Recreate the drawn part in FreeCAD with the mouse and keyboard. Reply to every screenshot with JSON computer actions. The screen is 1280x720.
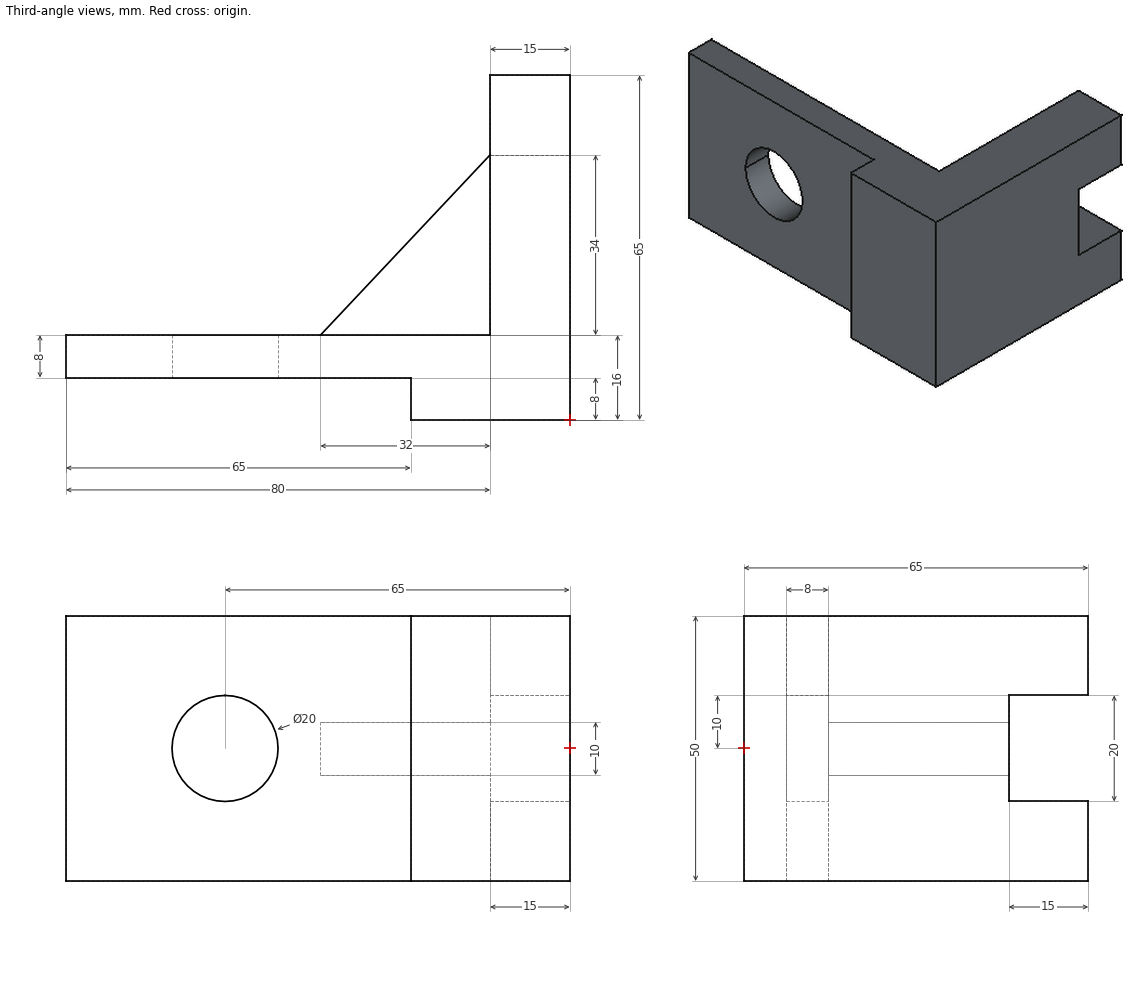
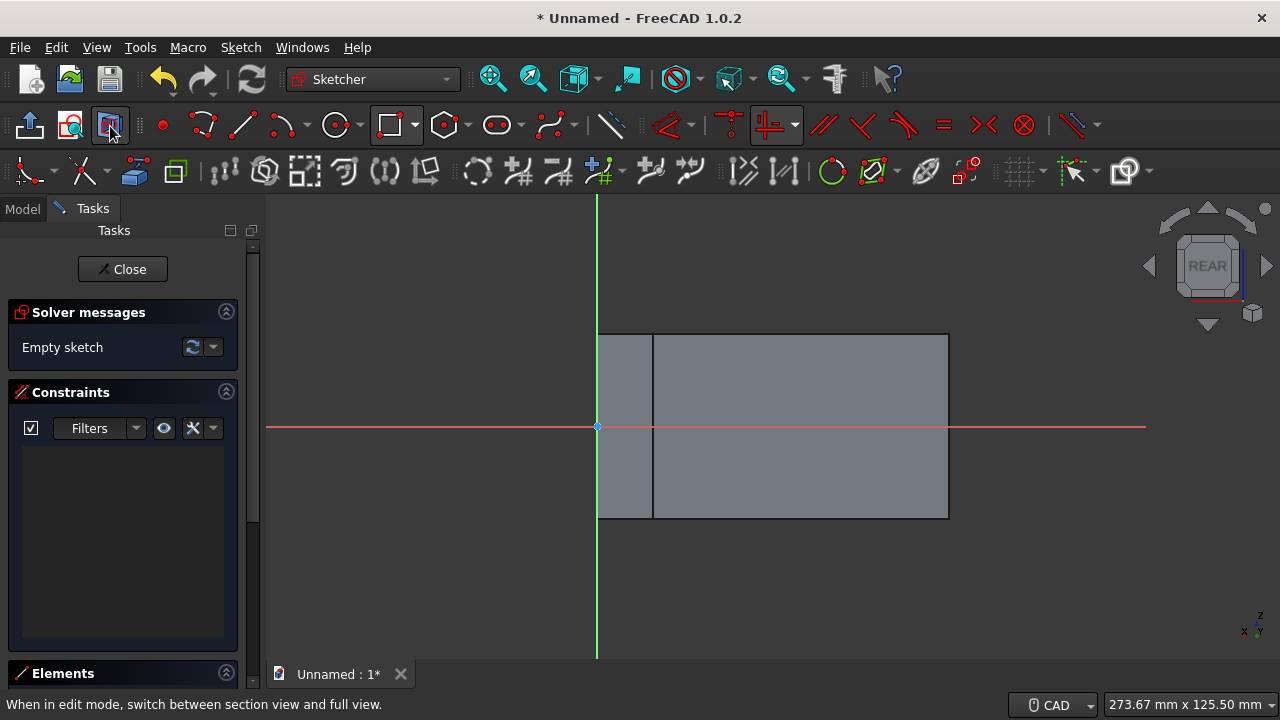
{"action": "scroll", "coordinate": [881, 426], "scroll_direction": "up", "scroll_amount": 7}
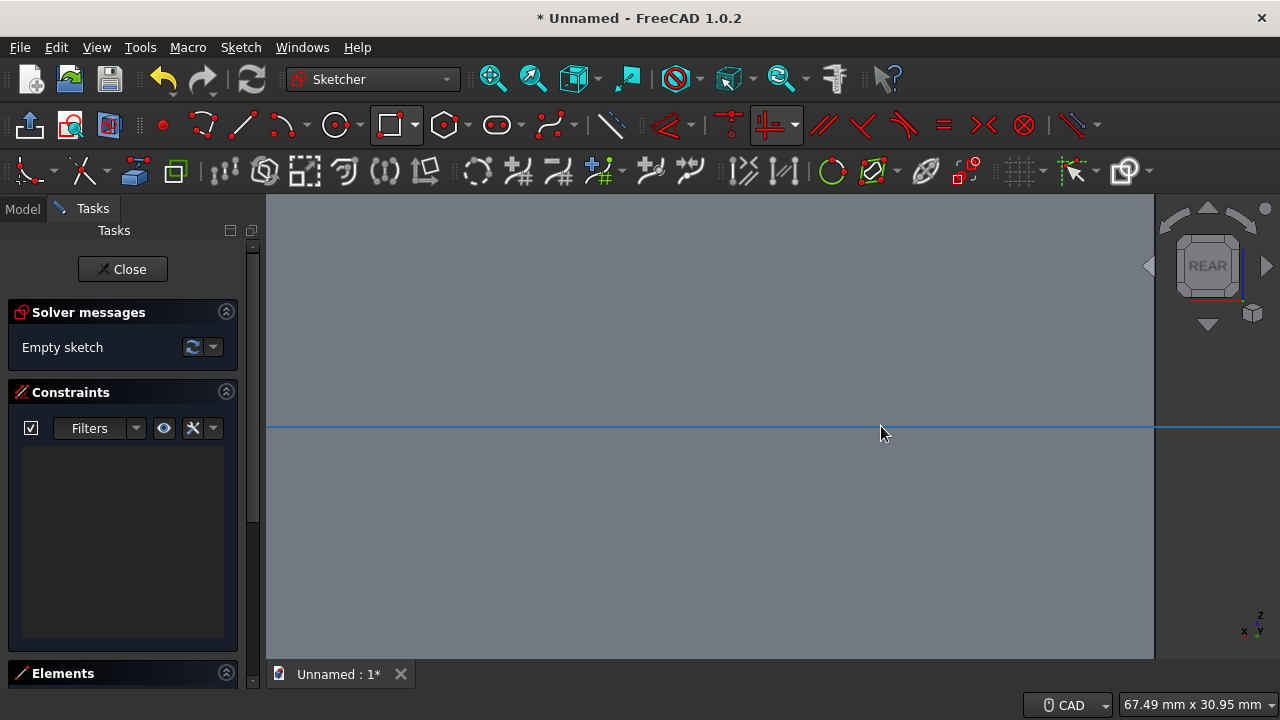
{"action": "key", "text": "g c"}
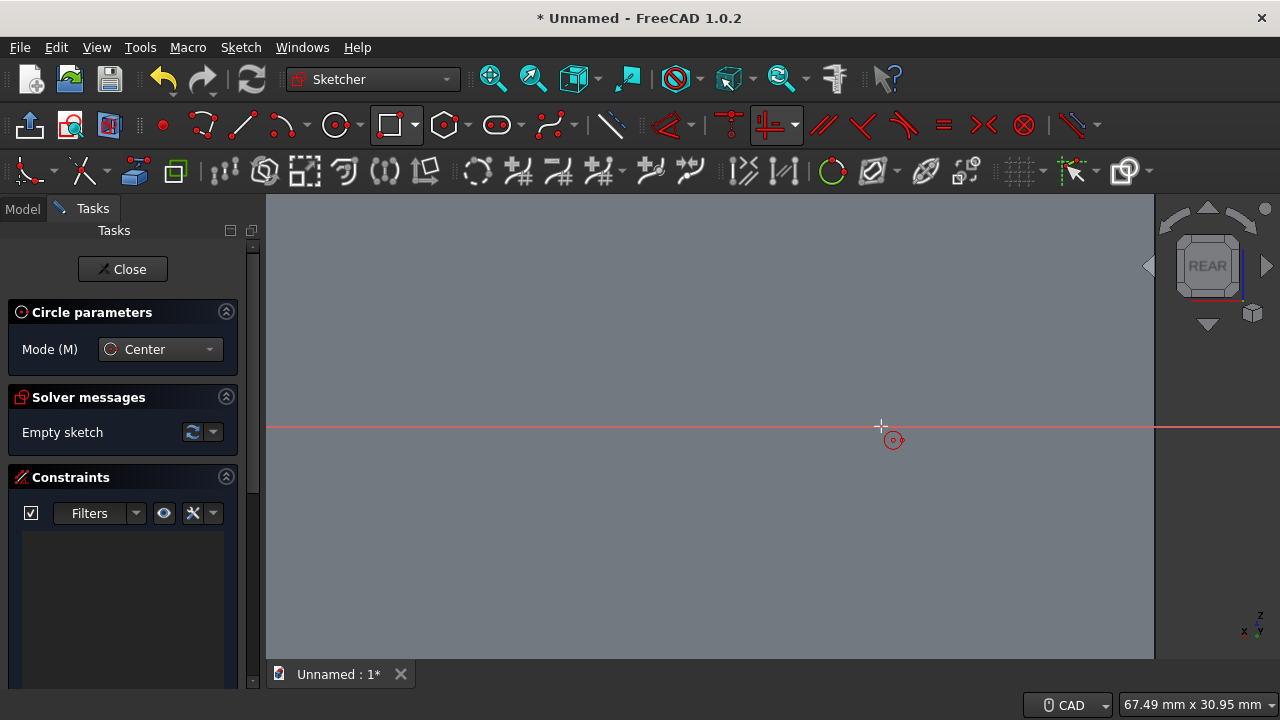
{"action": "left_click", "coordinate": [704, 426]}
{"action": "mouse_move", "coordinate": [810, 320]}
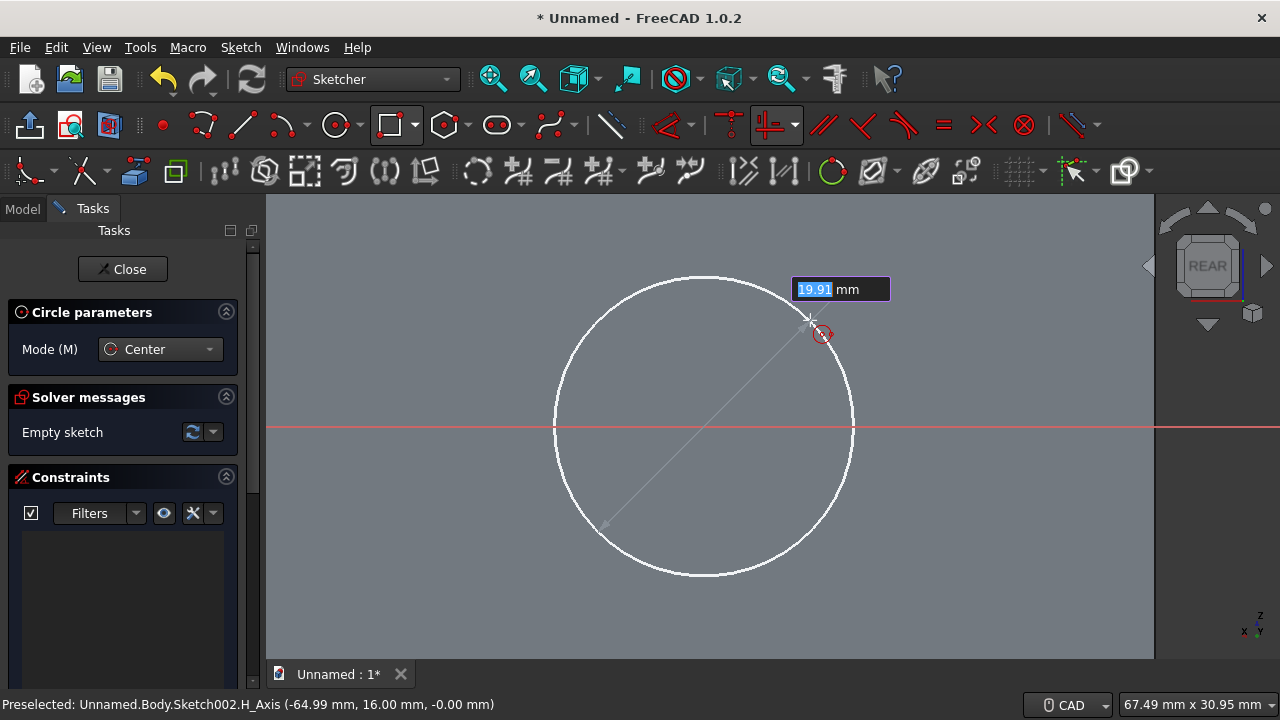
{"action": "type", "text": "20"}
{"action": "key", "text": "Return"}
{"action": "key", "text": "Escape"}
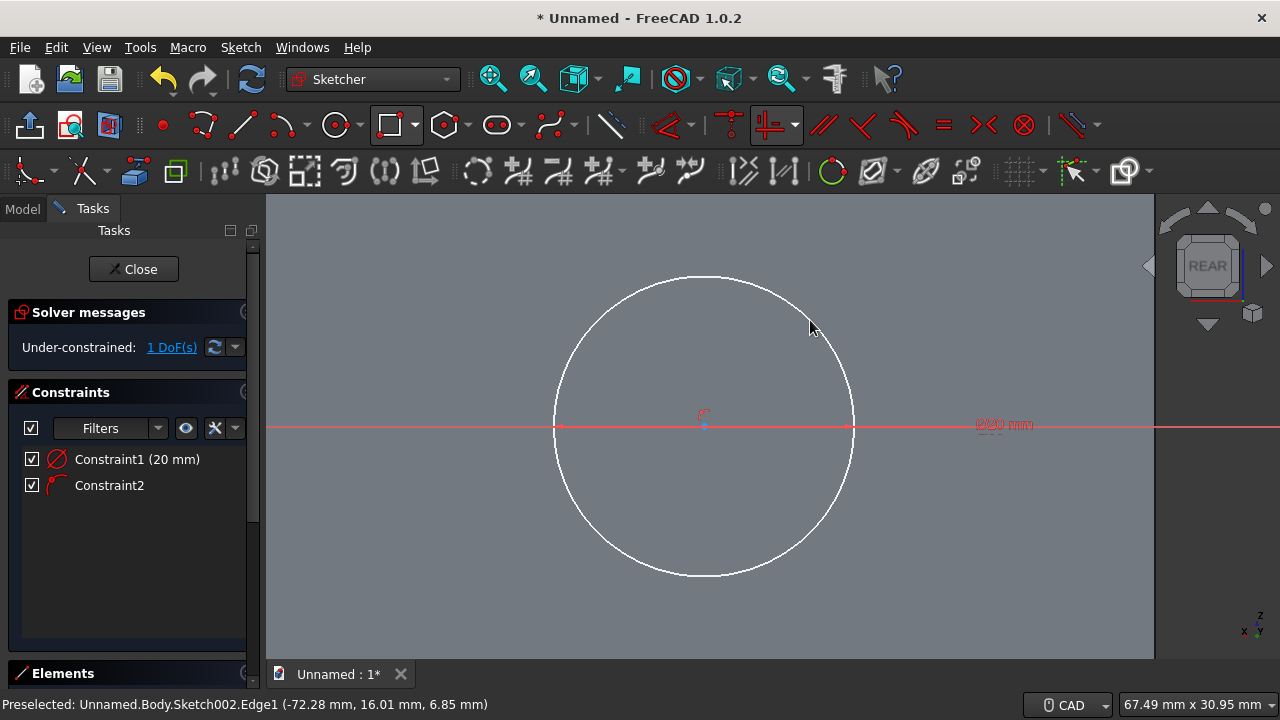
{"action": "key", "text": "d"}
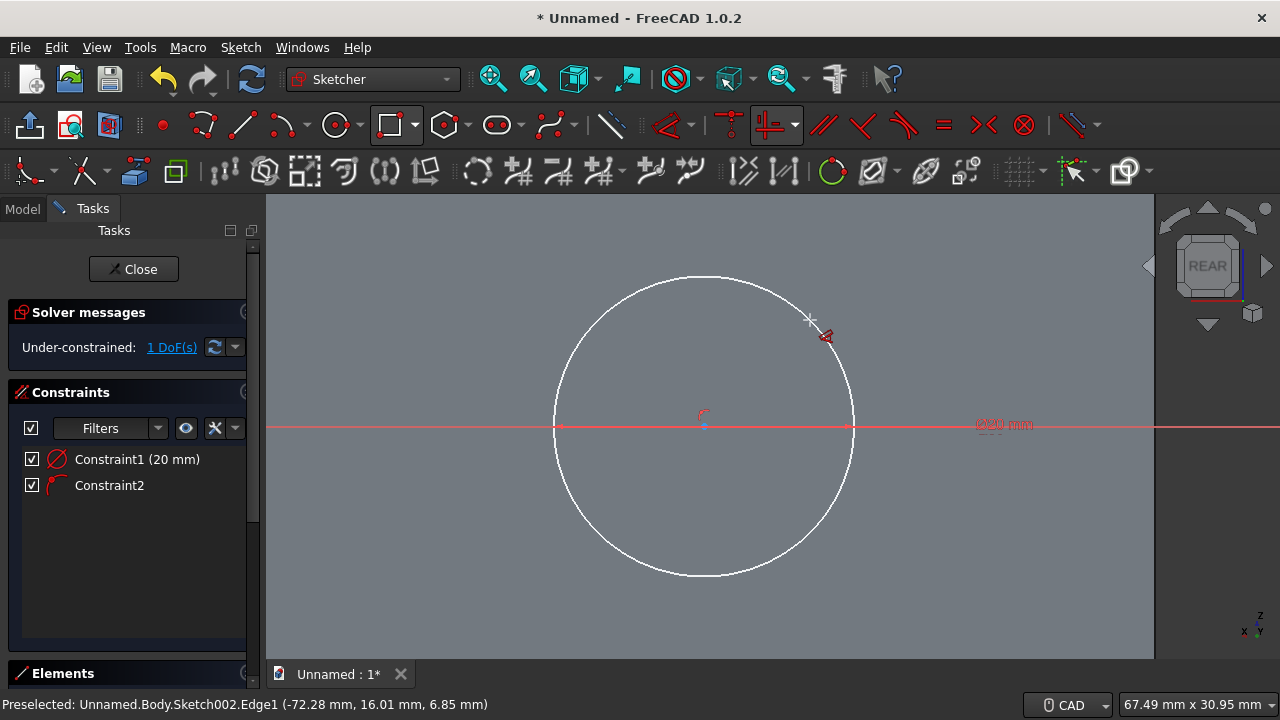
{"action": "left_click", "coordinate": [704, 426]}
{"action": "left_click", "coordinate": [499, 460]}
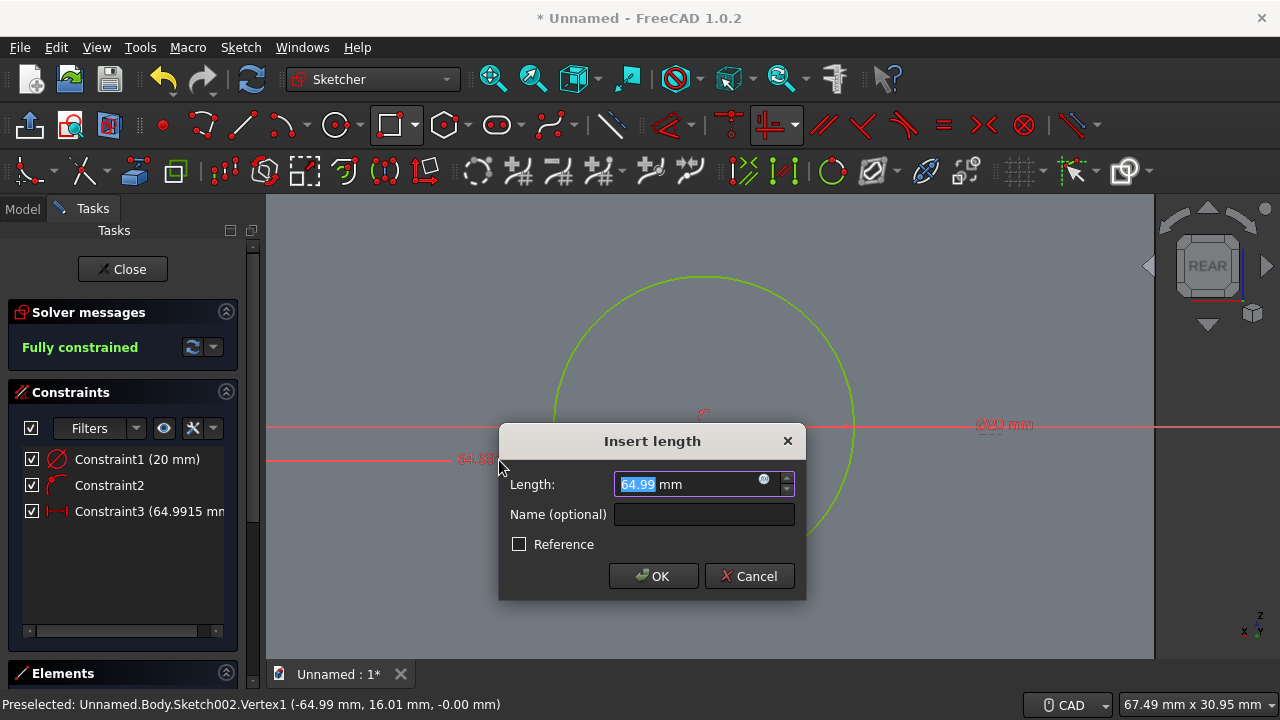
{"action": "type", "text": "65"}
{"action": "key", "text": "Return"}
{"action": "key", "text": "Escape"}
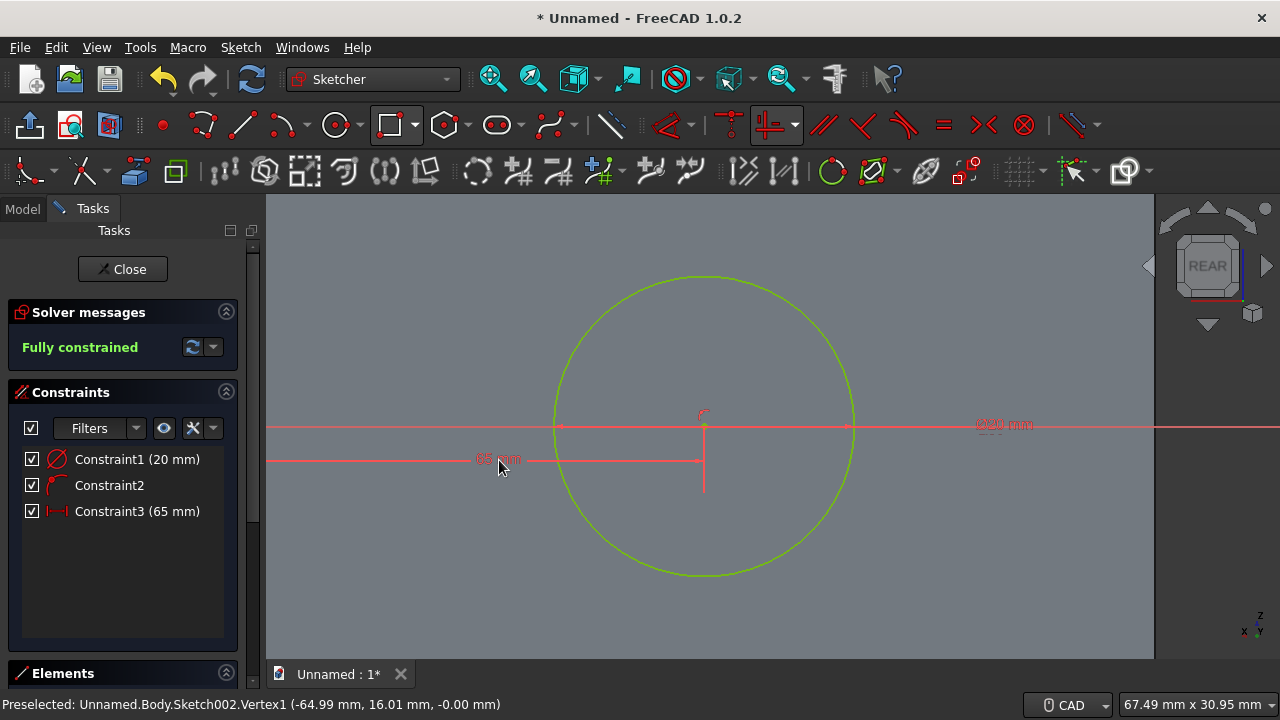
{"action": "left_click", "coordinate": [123, 269]}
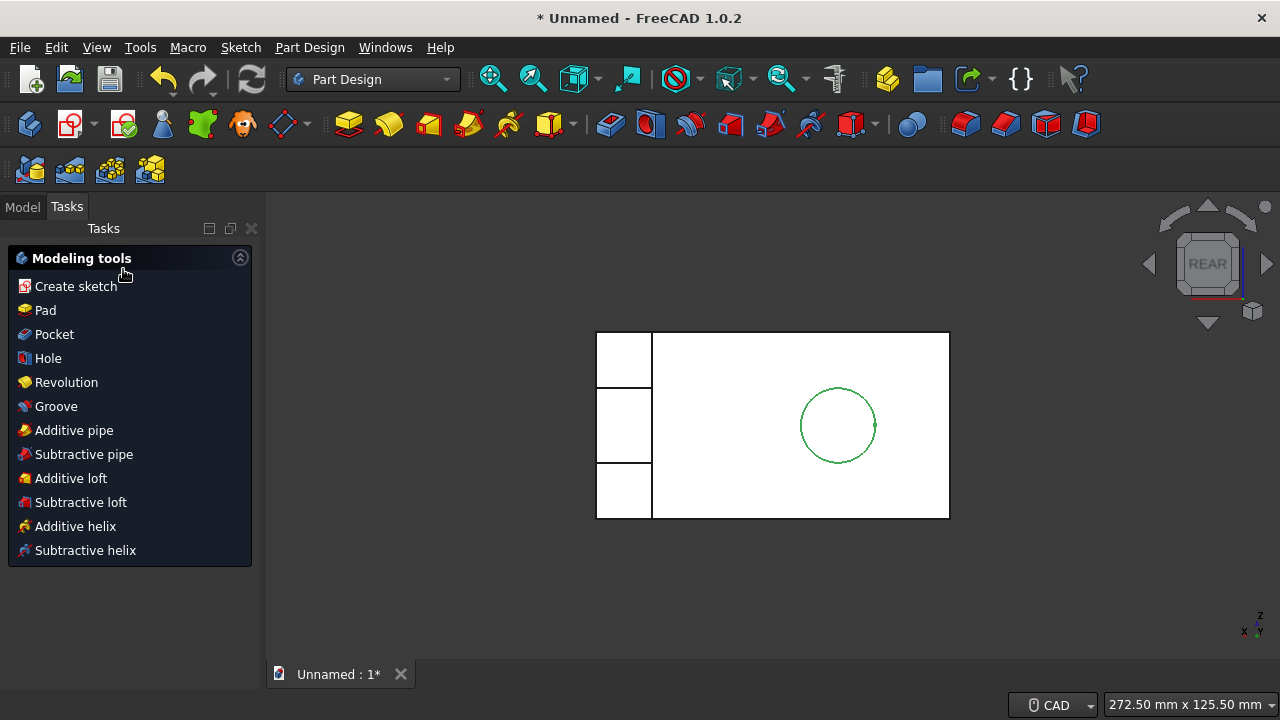
{"action": "left_click", "coordinate": [612, 124]}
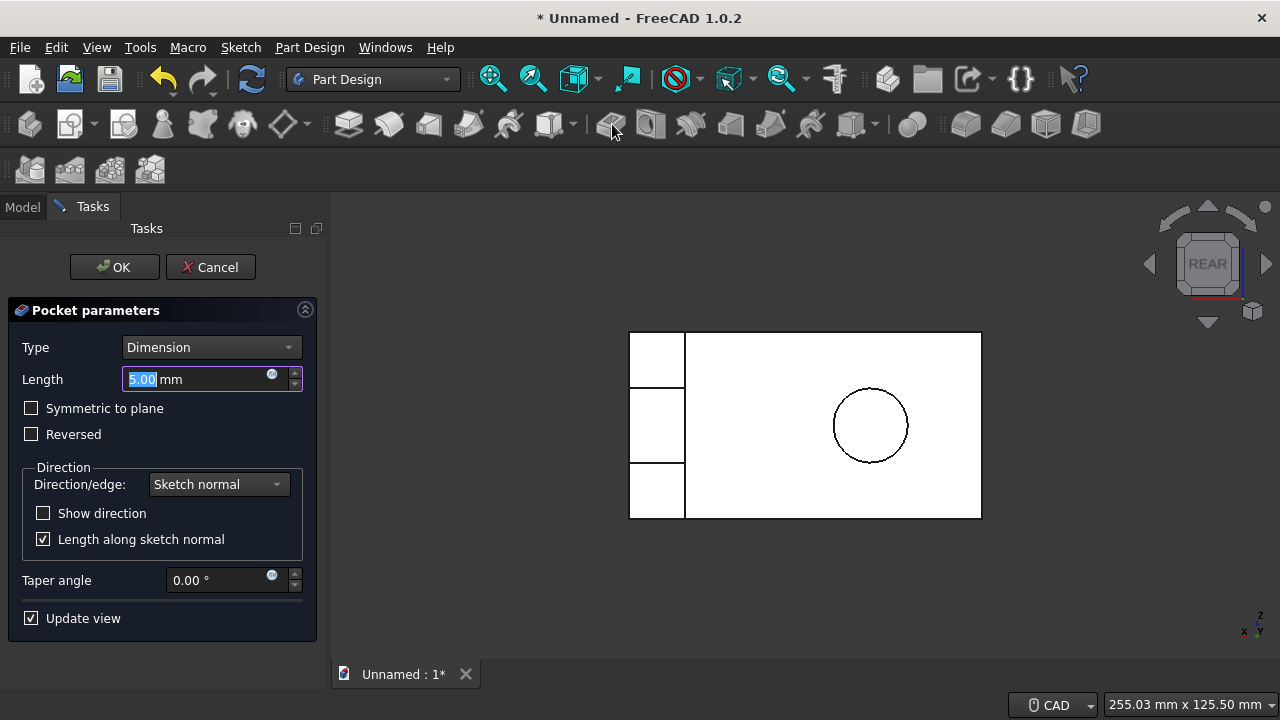
{"action": "type", "text": "8"}
{"action": "key", "text": "Tab"}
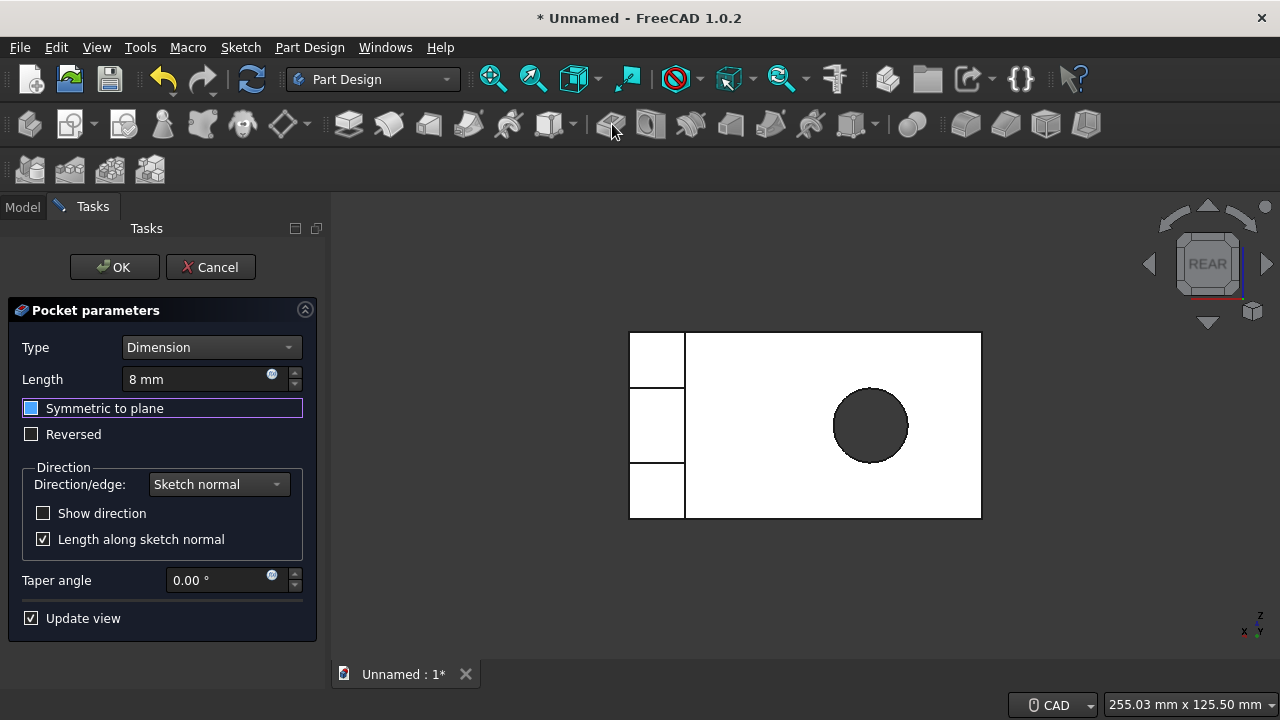
{"action": "left_click", "coordinate": [115, 267]}